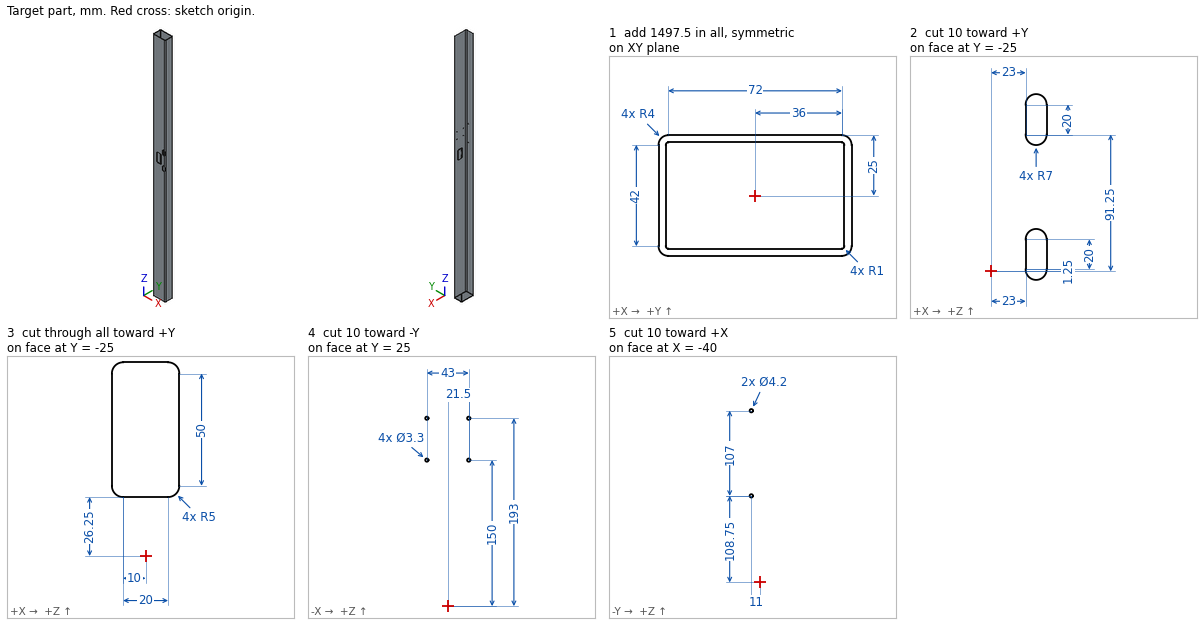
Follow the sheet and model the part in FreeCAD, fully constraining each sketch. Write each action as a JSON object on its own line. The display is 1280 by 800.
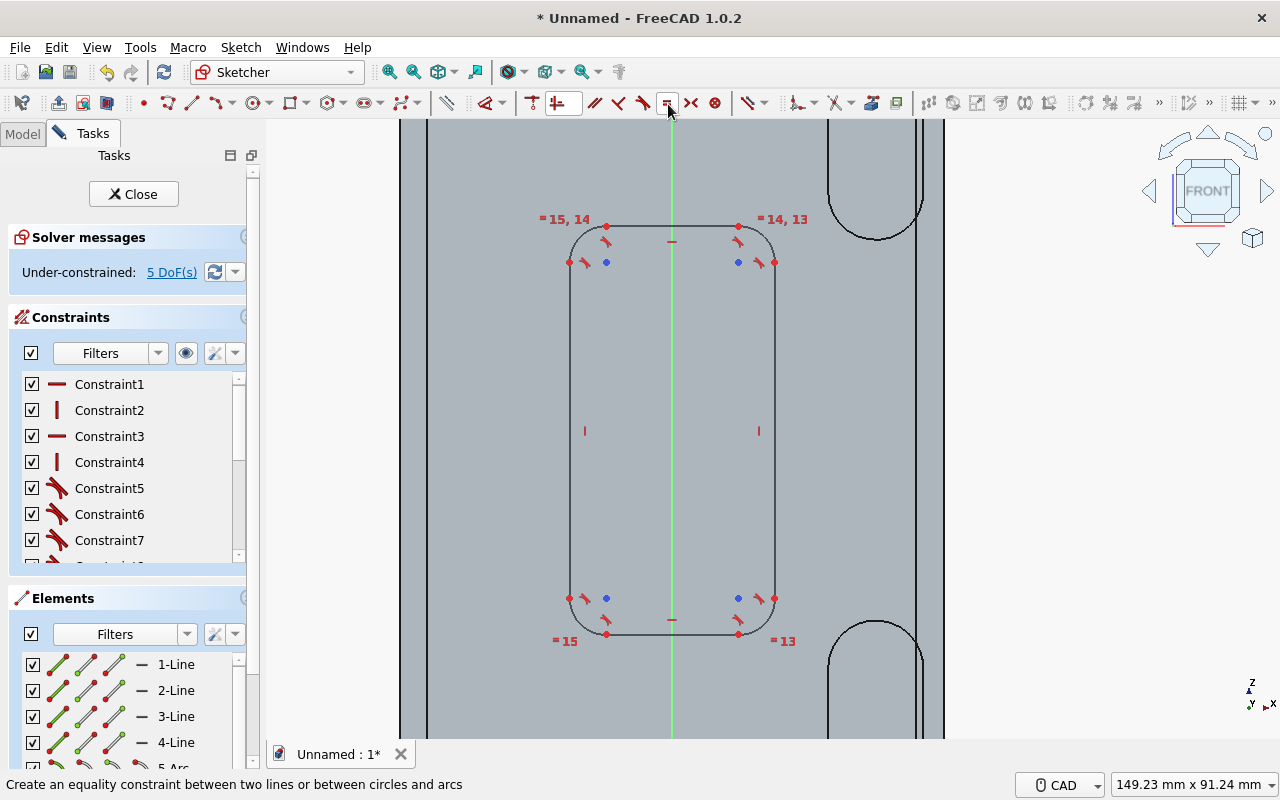
{"action": "key", "text": "d"}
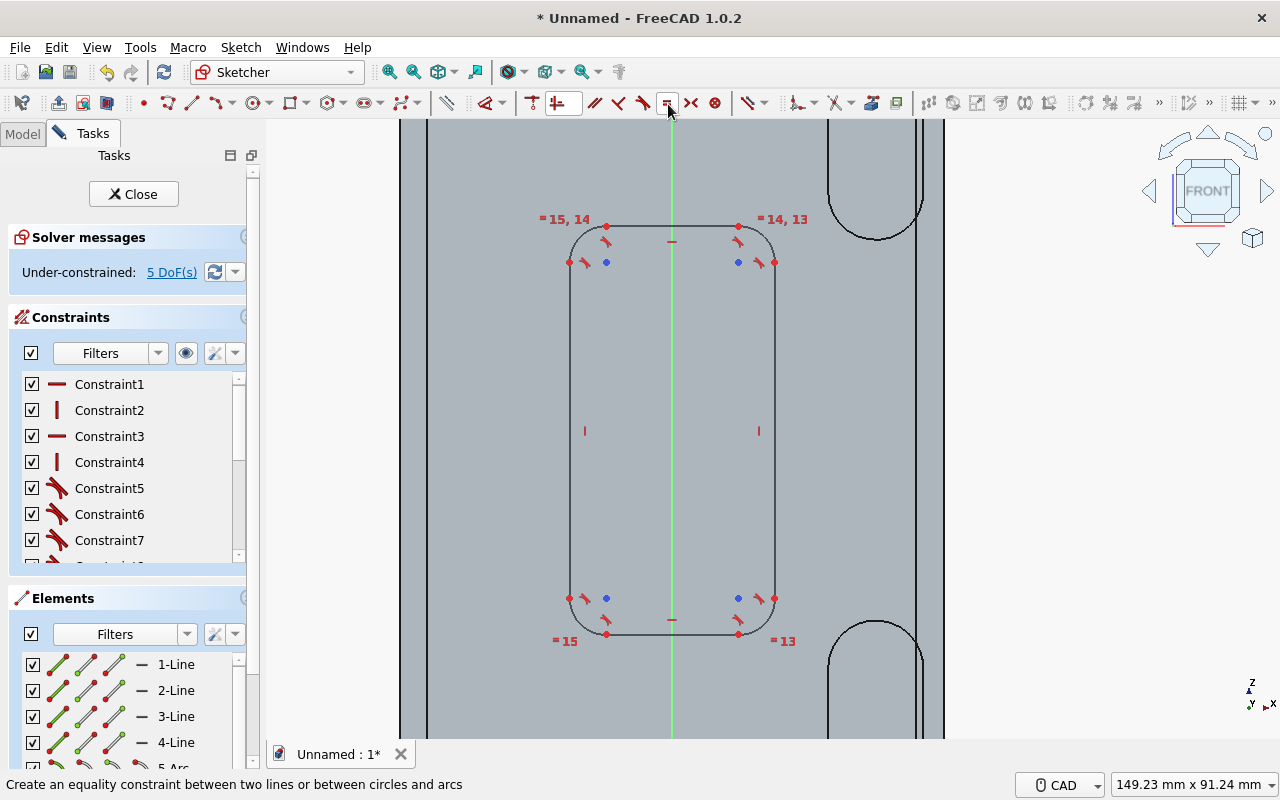
{"action": "left_click", "coordinate": [755, 631]}
{"action": "left_click", "coordinate": [769, 660]}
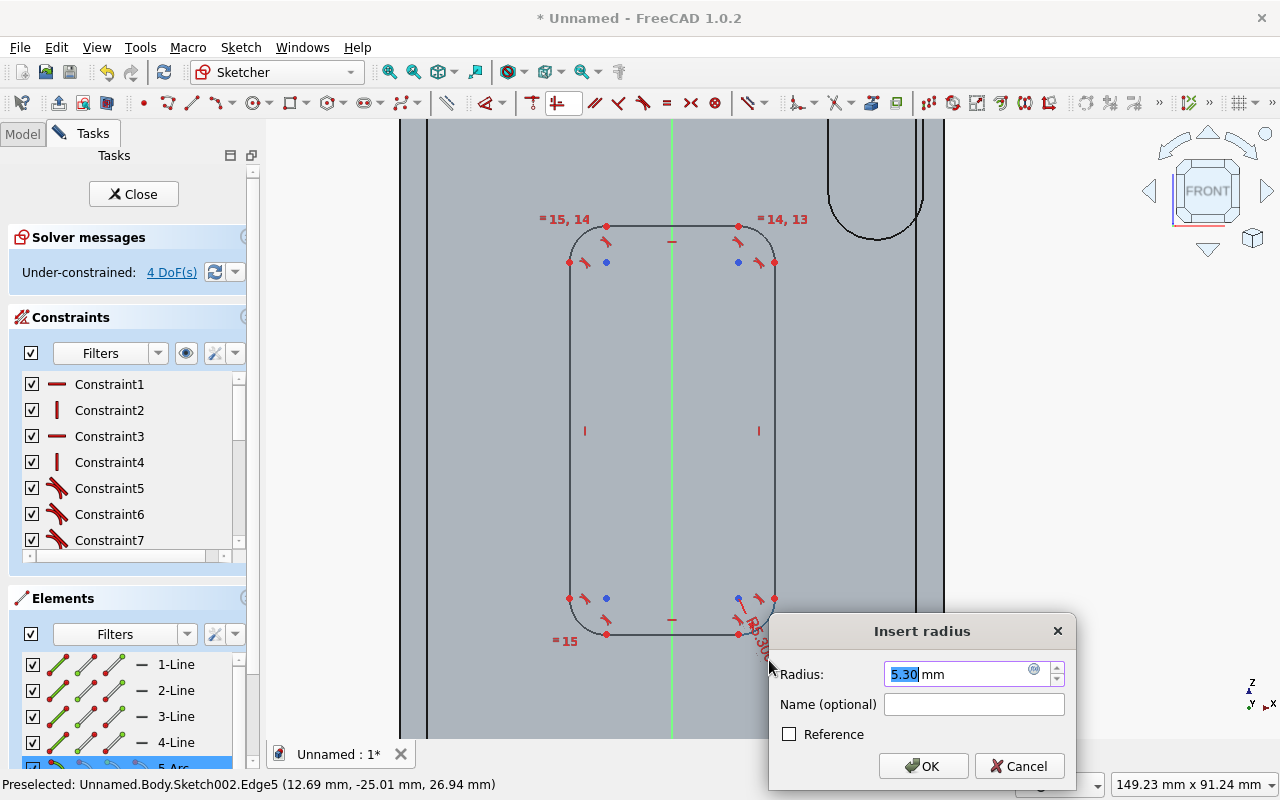
{"action": "type", "text": "5"}
{"action": "key", "text": "Return"}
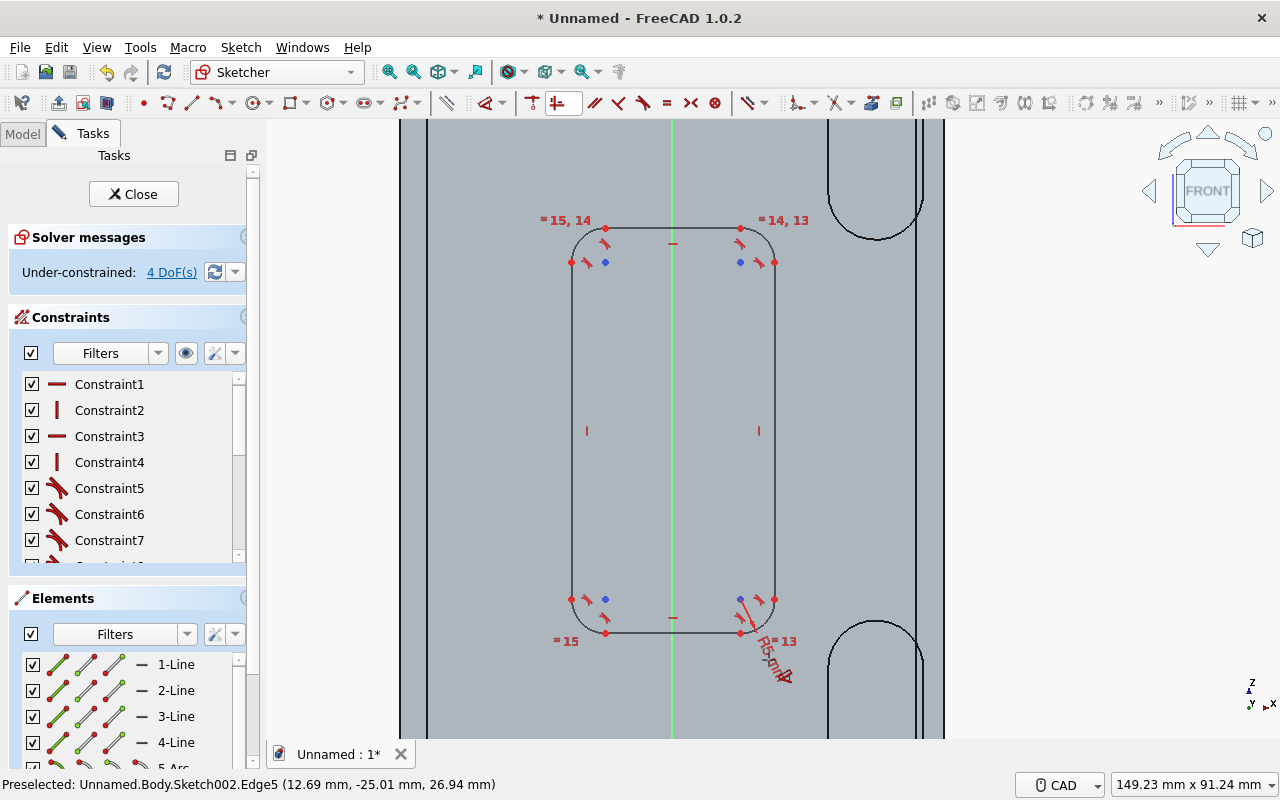
{"action": "left_click", "coordinate": [646, 633]}
{"action": "left_click", "coordinate": [642, 667]}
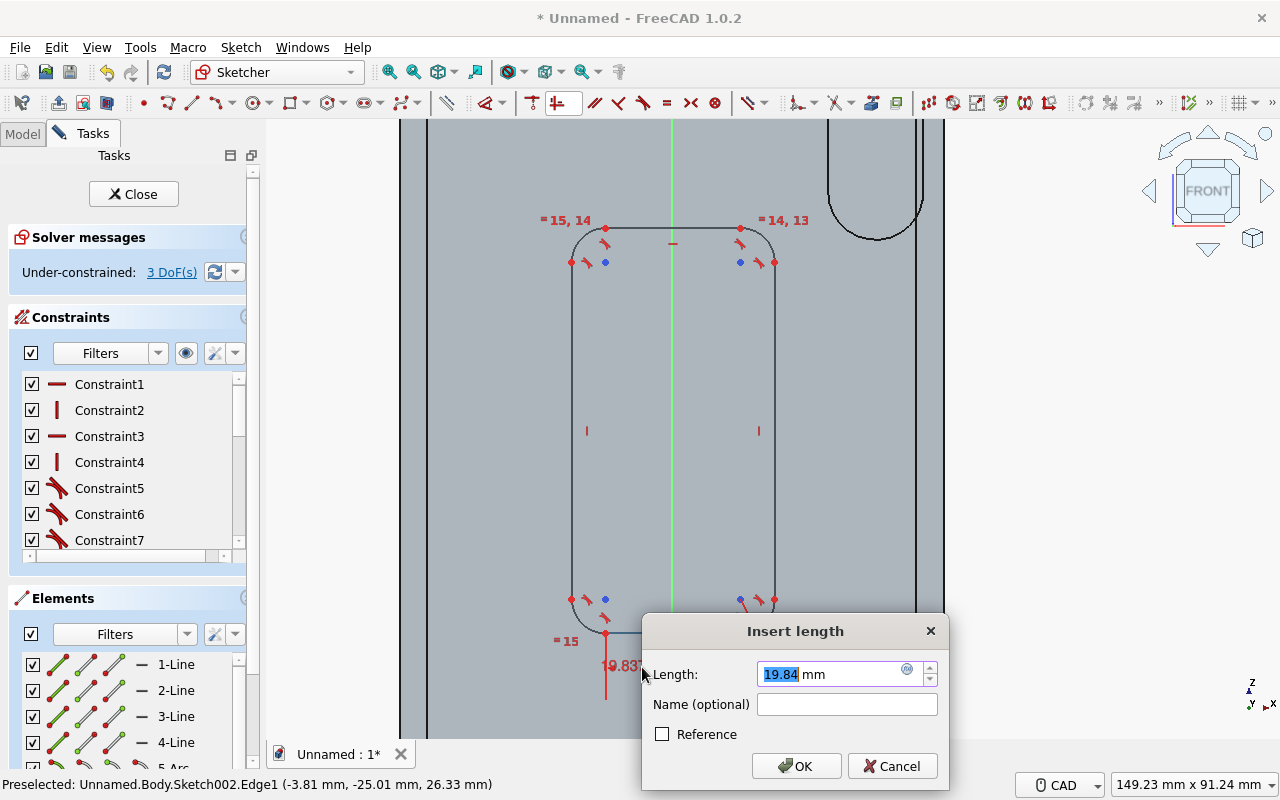
{"action": "type", "text": "20"}
{"action": "key", "text": "Return"}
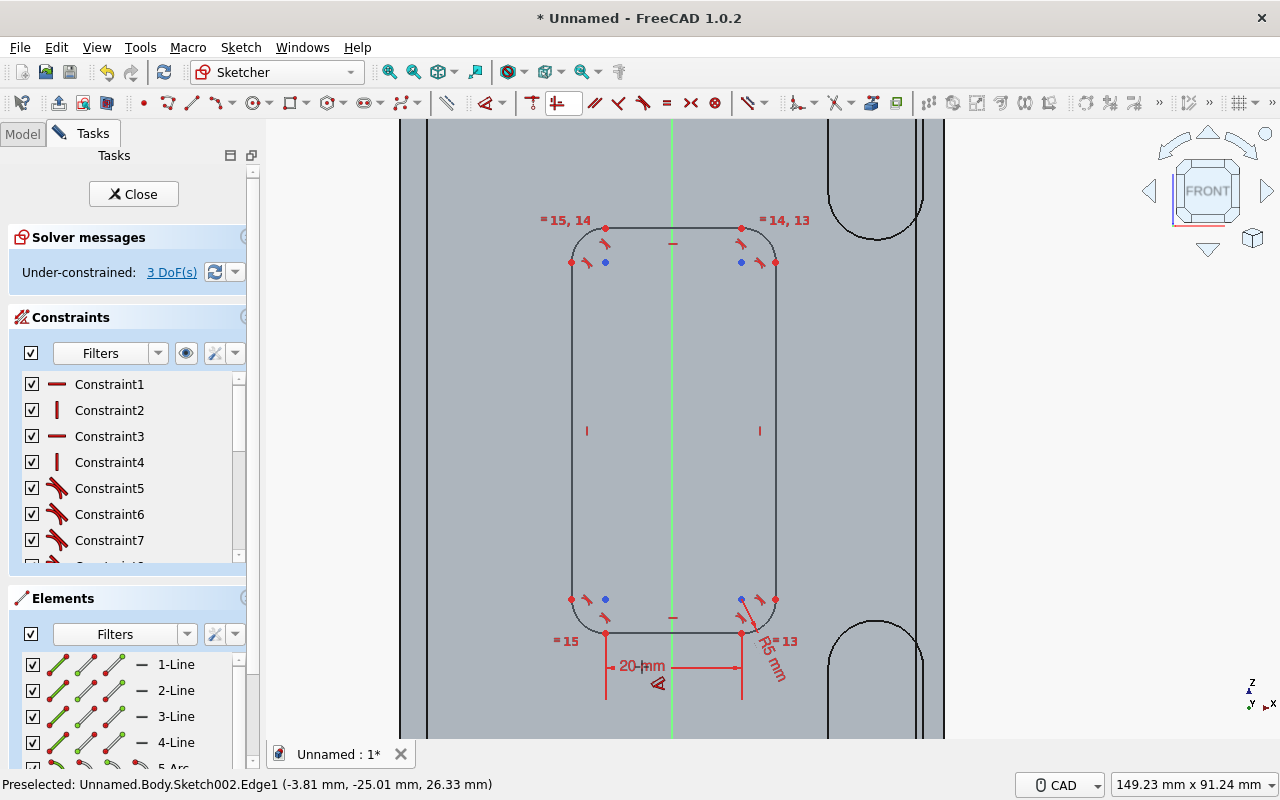
{"action": "left_click", "coordinate": [776, 498]}
{"action": "left_click", "coordinate": [810, 431]}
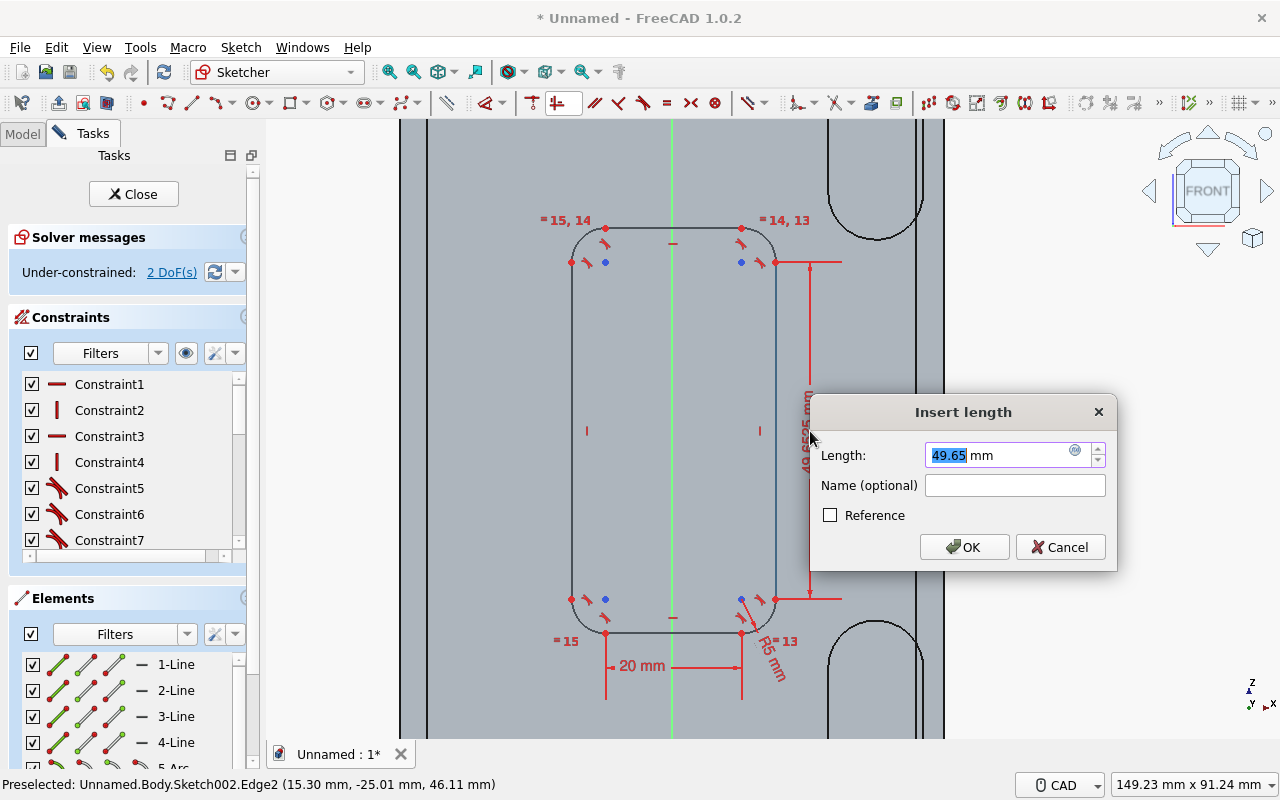
{"action": "type", "text": "50"}
{"action": "key", "text": "Return"}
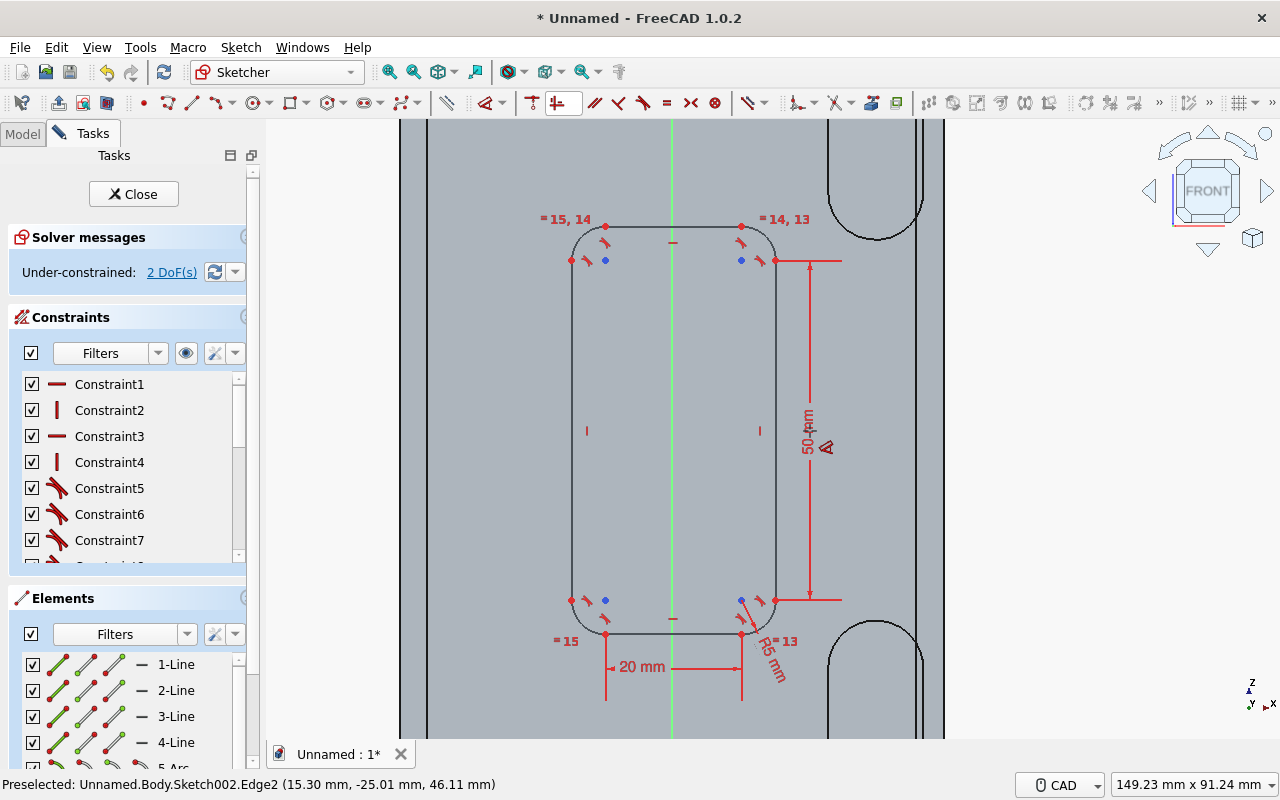
{"action": "left_click", "coordinate": [606, 634]}
{"action": "left_click", "coordinate": [639, 600]}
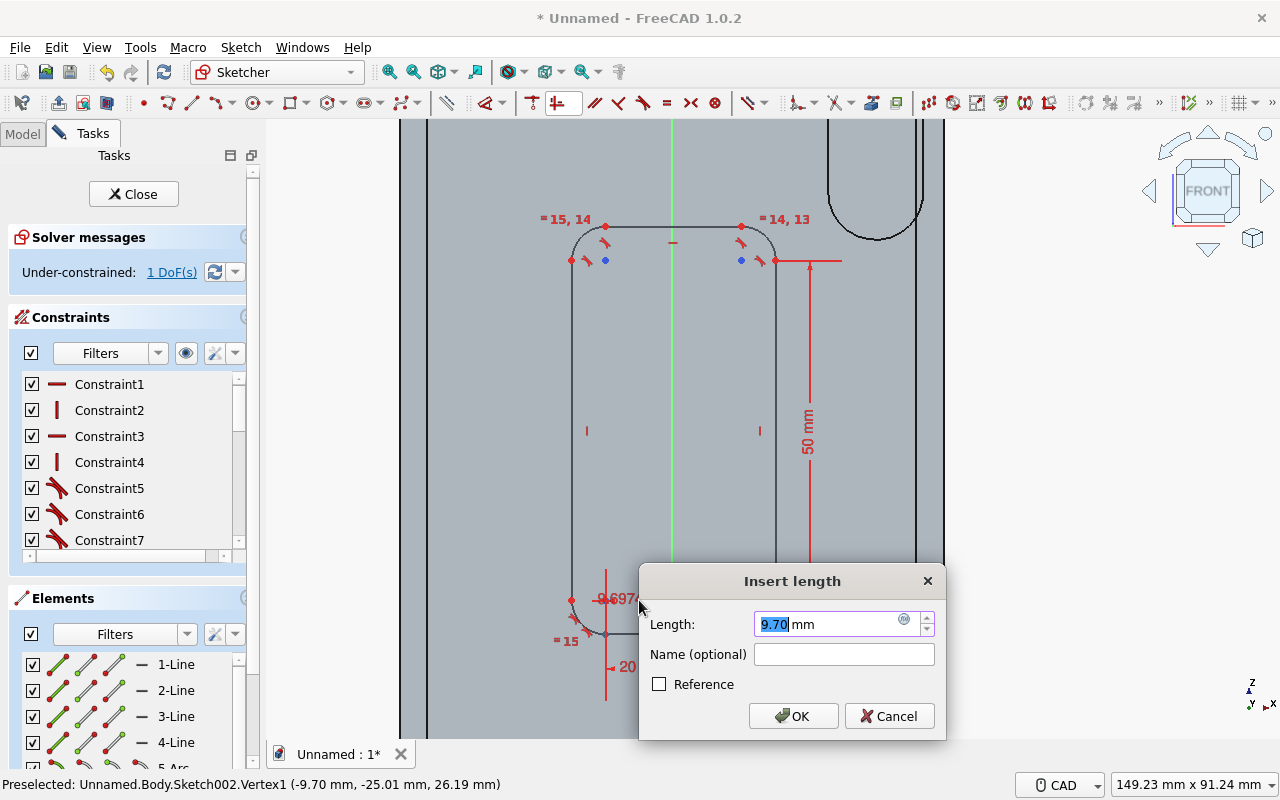
{"action": "type", "text": "10"}
{"action": "key", "text": "Return"}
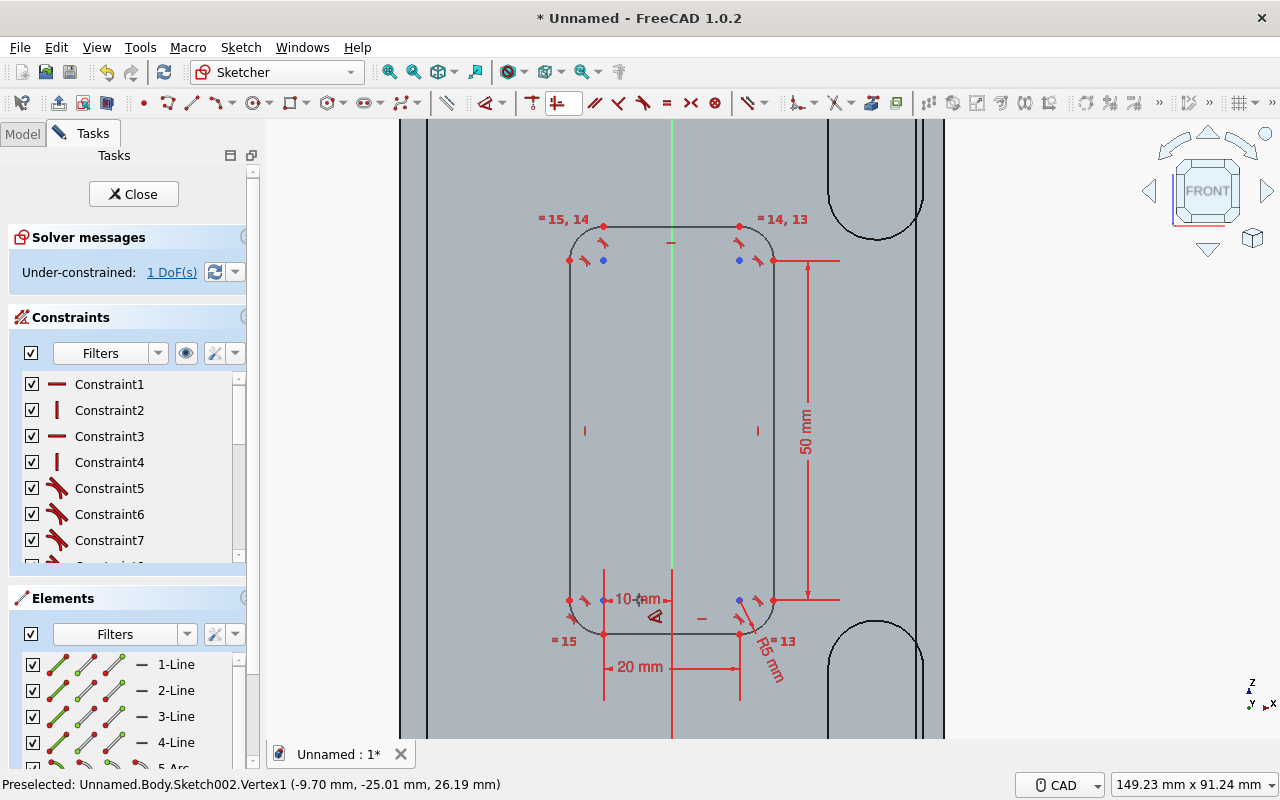
{"action": "left_click", "coordinate": [604, 634]}
{"action": "left_click", "coordinate": [570, 673]}